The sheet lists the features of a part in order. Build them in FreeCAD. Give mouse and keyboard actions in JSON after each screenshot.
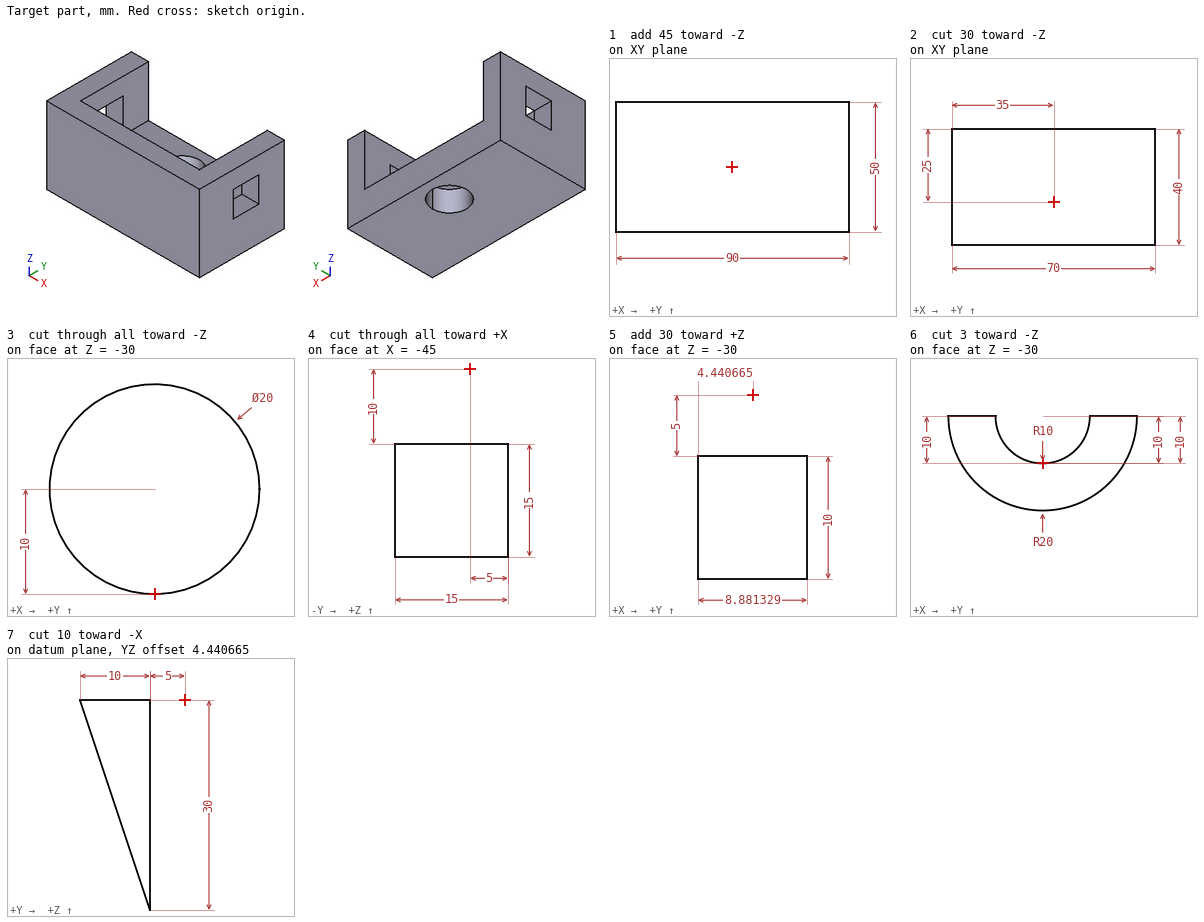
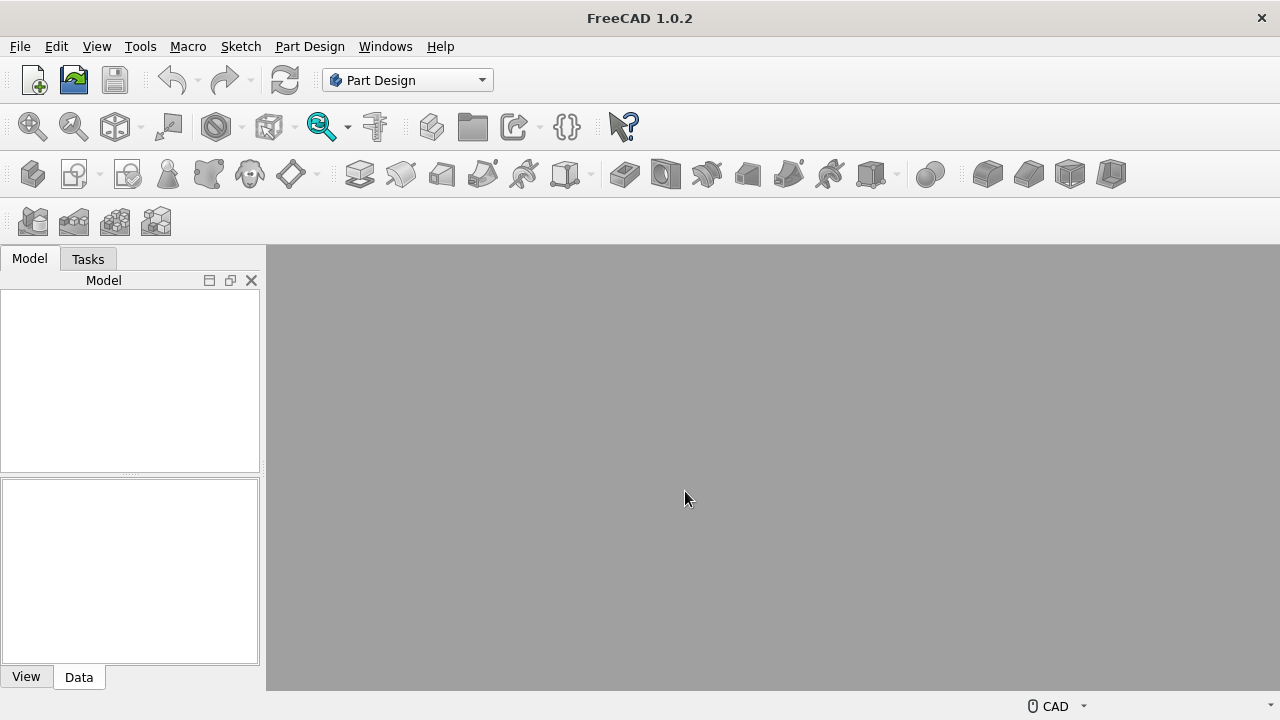
{"action": "key", "text": "ctrl+n"}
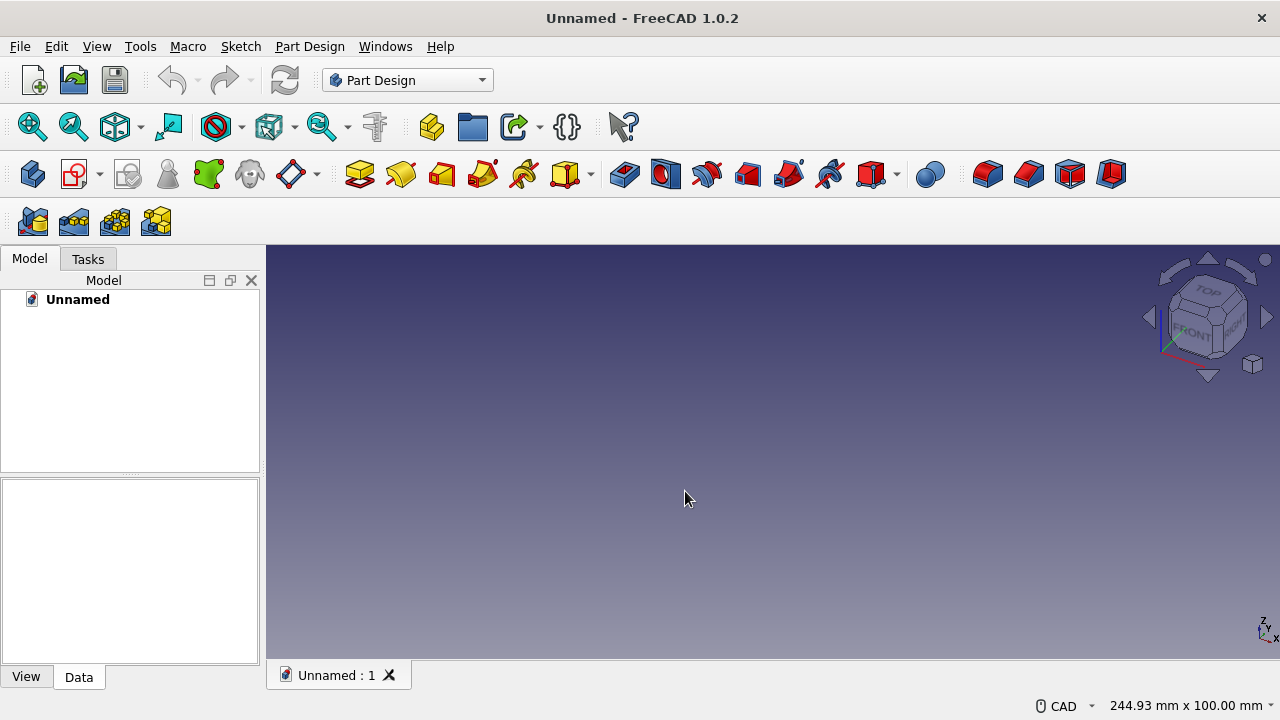
{"action": "left_click", "coordinate": [74, 174]}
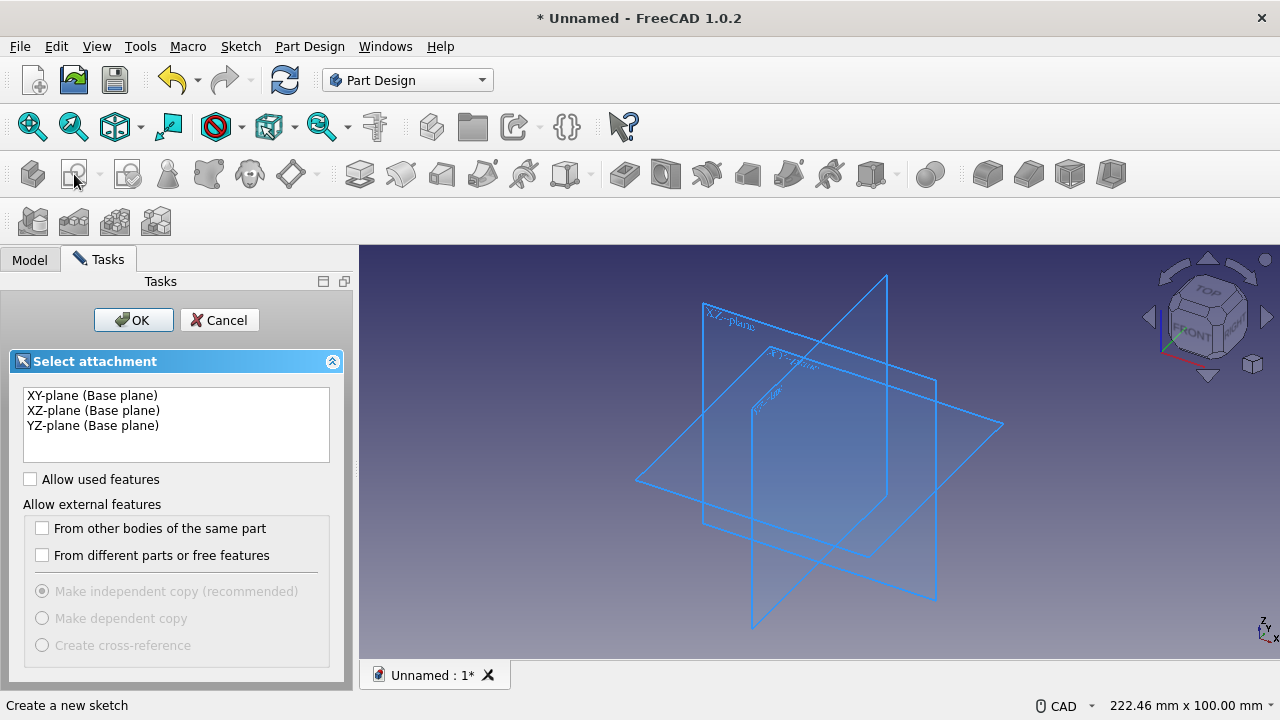
{"action": "left_click", "coordinate": [84, 396]}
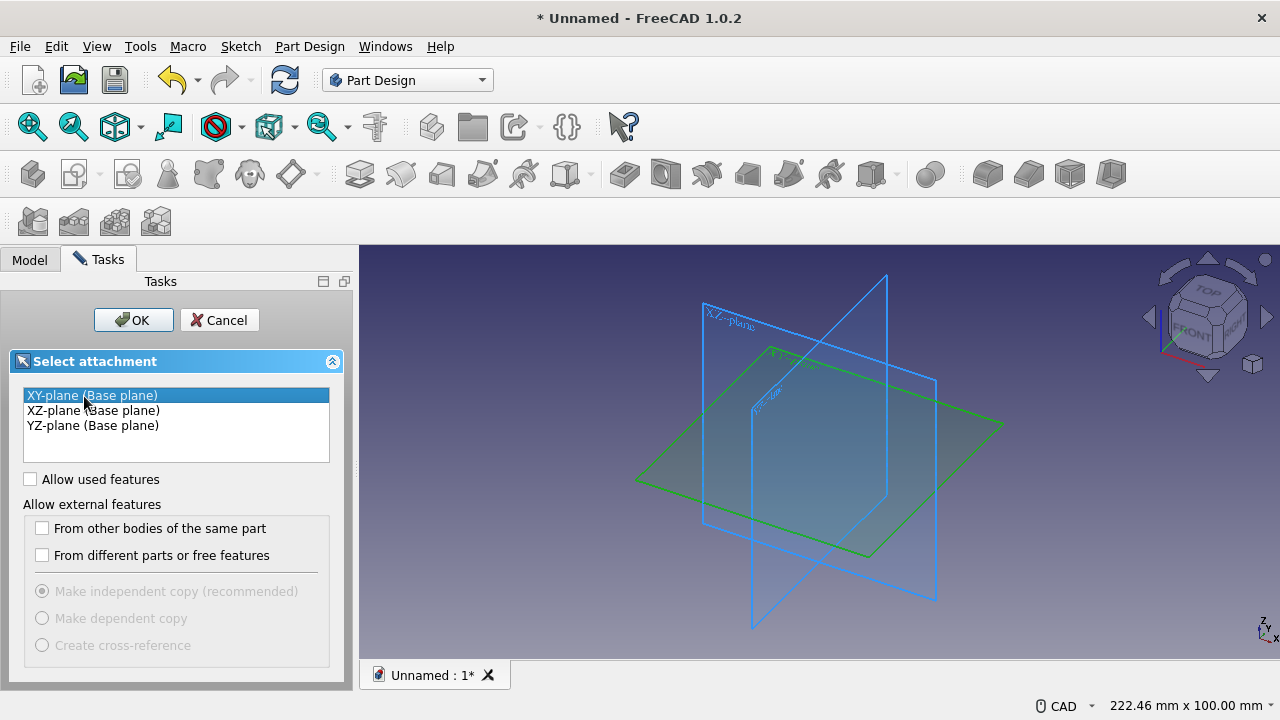
{"action": "left_click", "coordinate": [134, 320]}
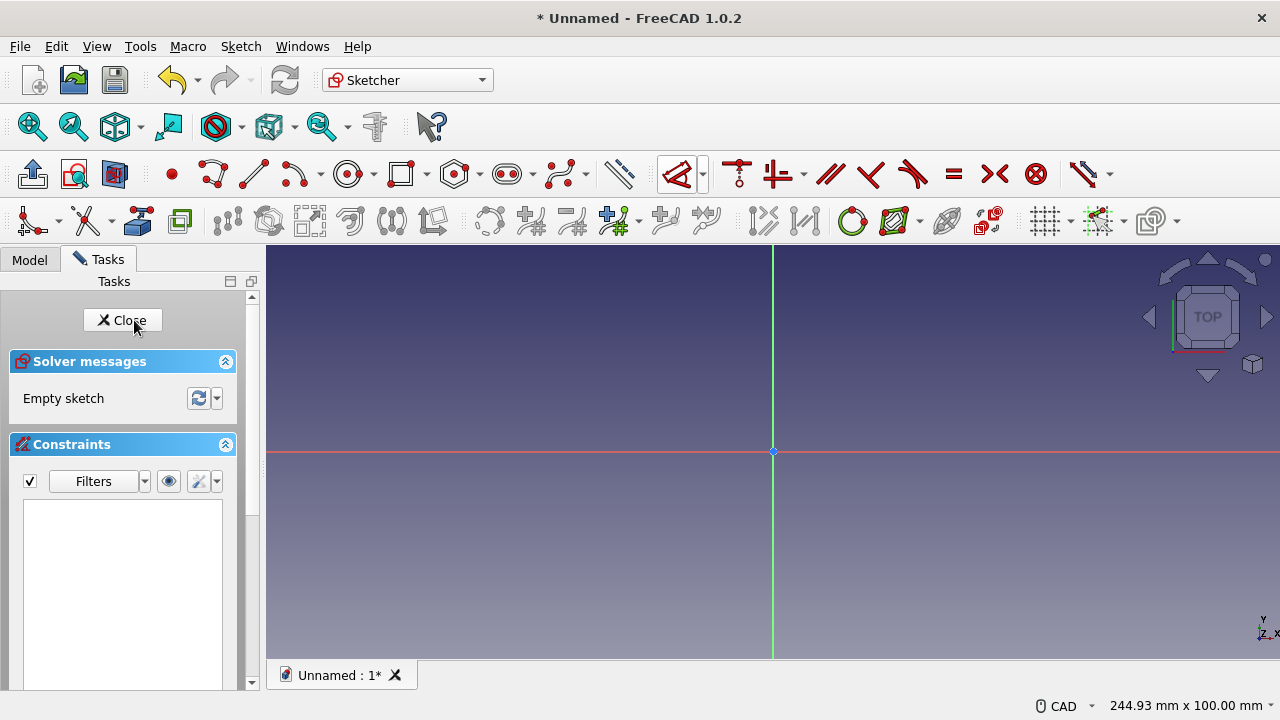
{"action": "key", "text": "g v"}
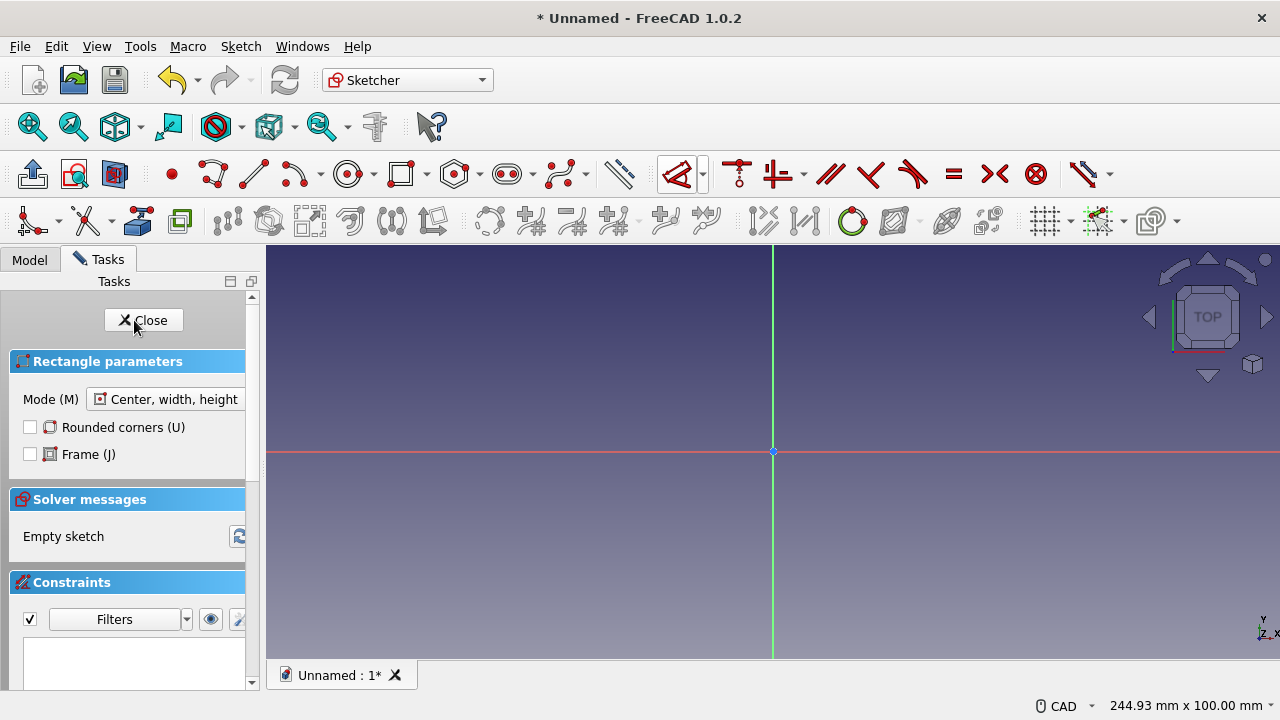
{"action": "left_click", "coordinate": [773, 452]}
{"action": "mouse_move", "coordinate": [959, 348]}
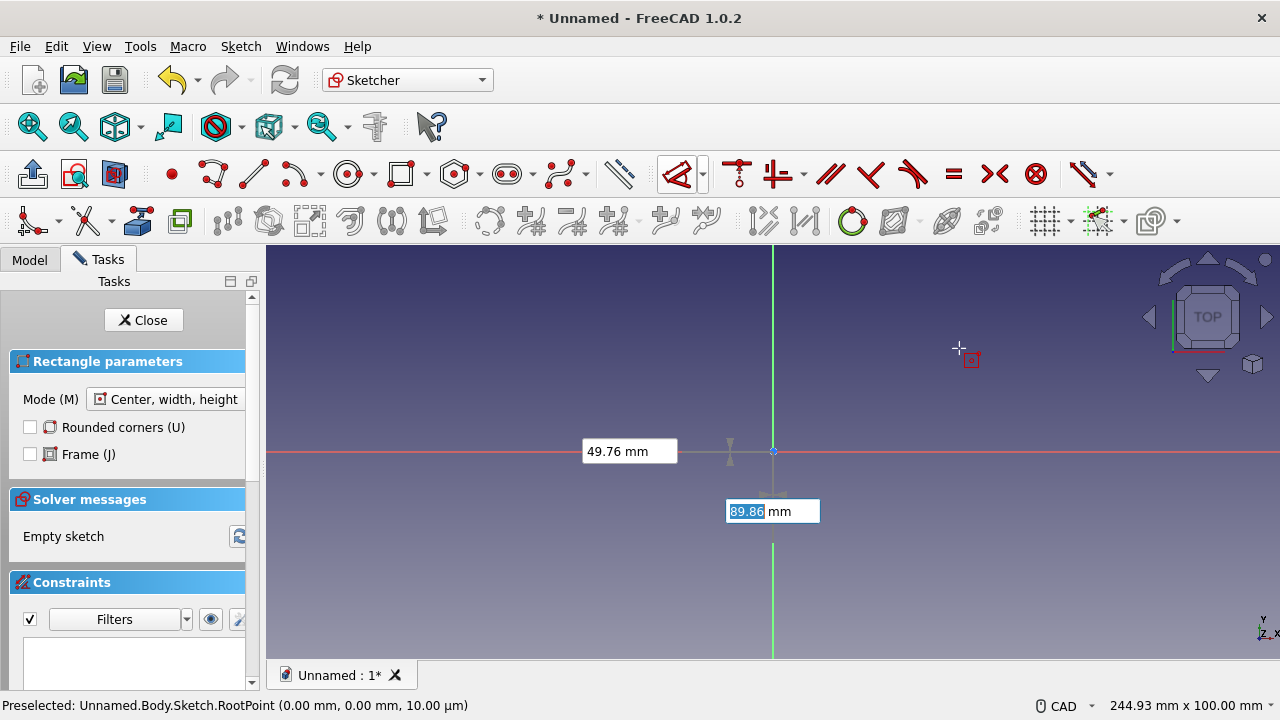
{"action": "type", "text": "90"}
{"action": "key", "text": "Tab"}
{"action": "type", "text": "50"}
{"action": "key", "text": "Return"}
{"action": "key", "text": "Escape"}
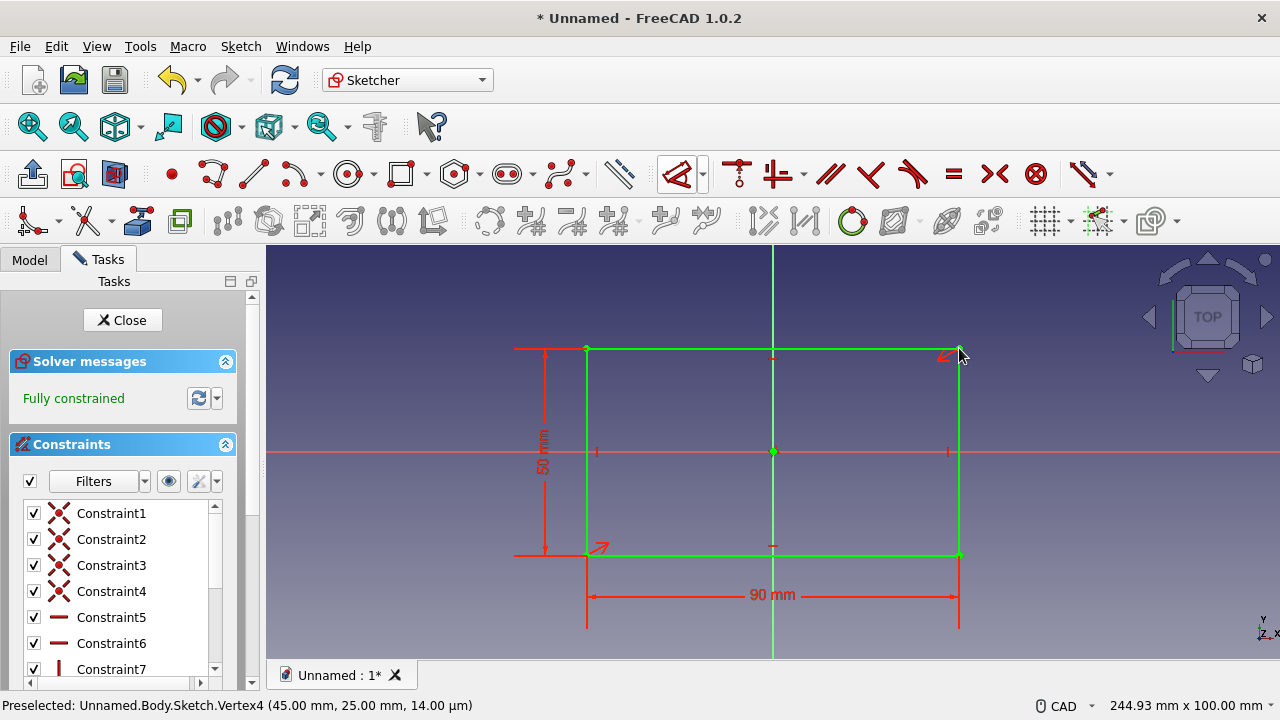
{"action": "left_click", "coordinate": [123, 320]}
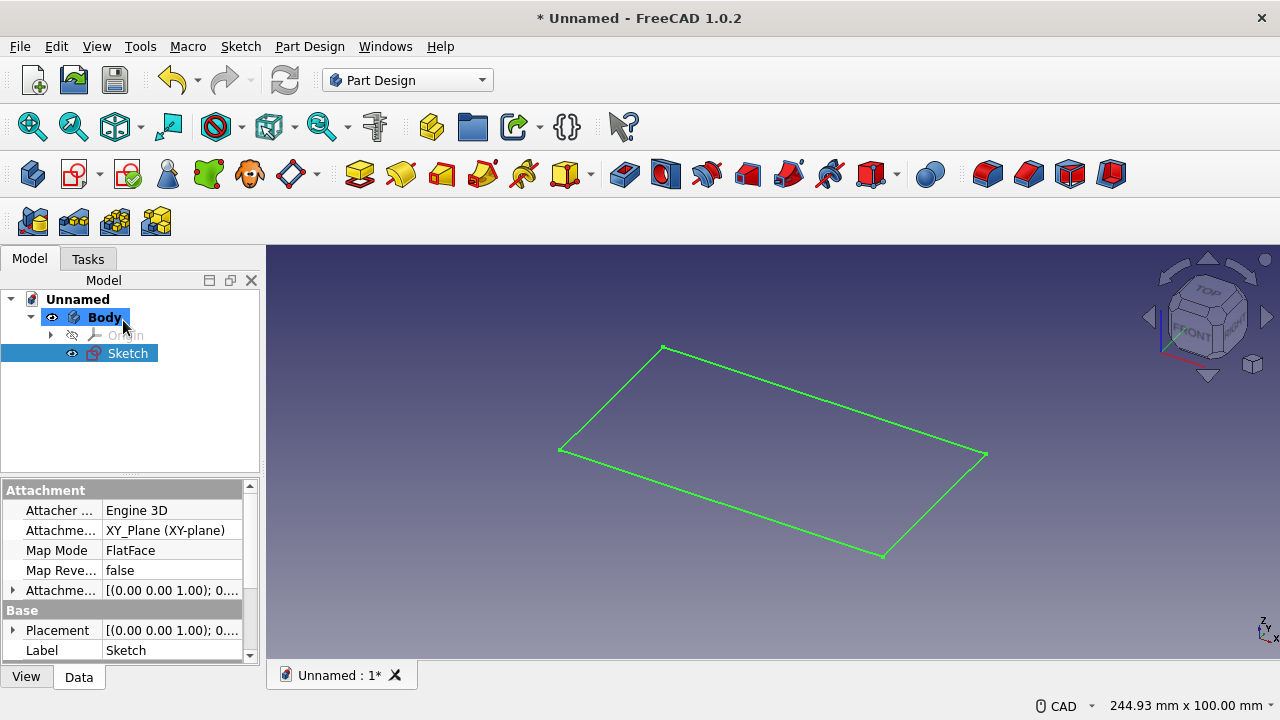
{"action": "left_click", "coordinate": [360, 174]}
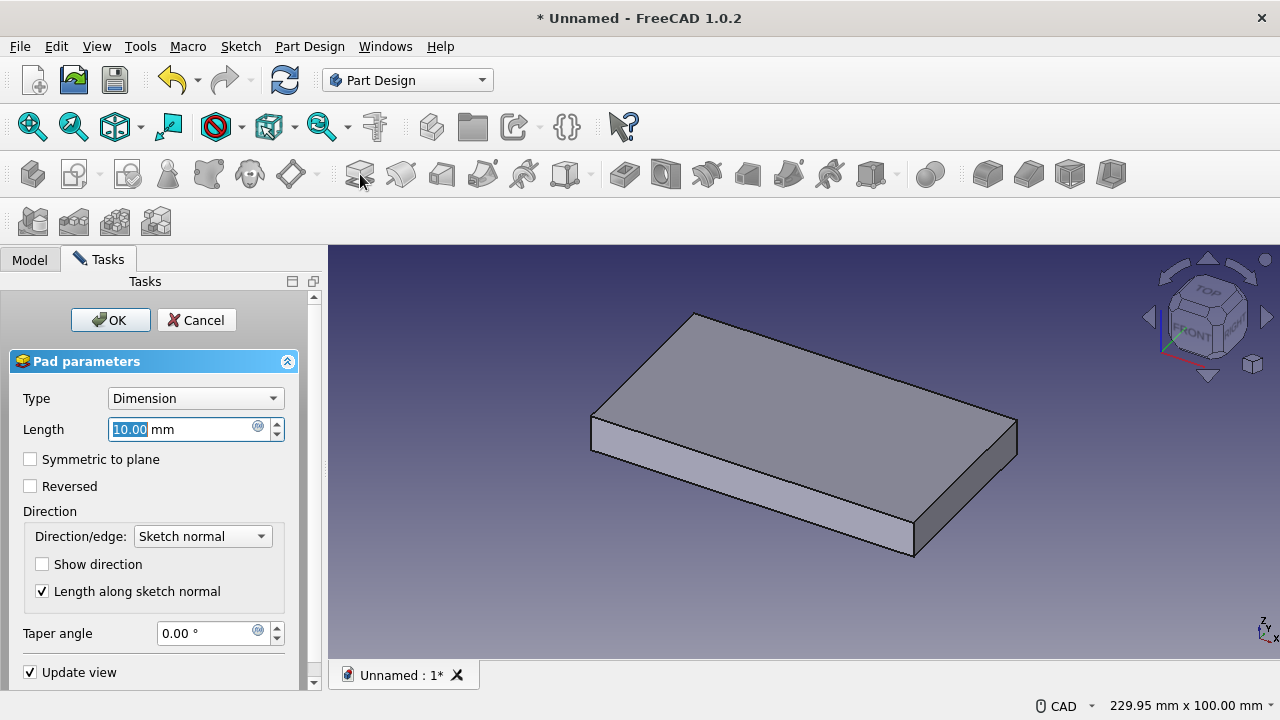
{"action": "type", "text": "45"}
{"action": "key", "text": "Tab"}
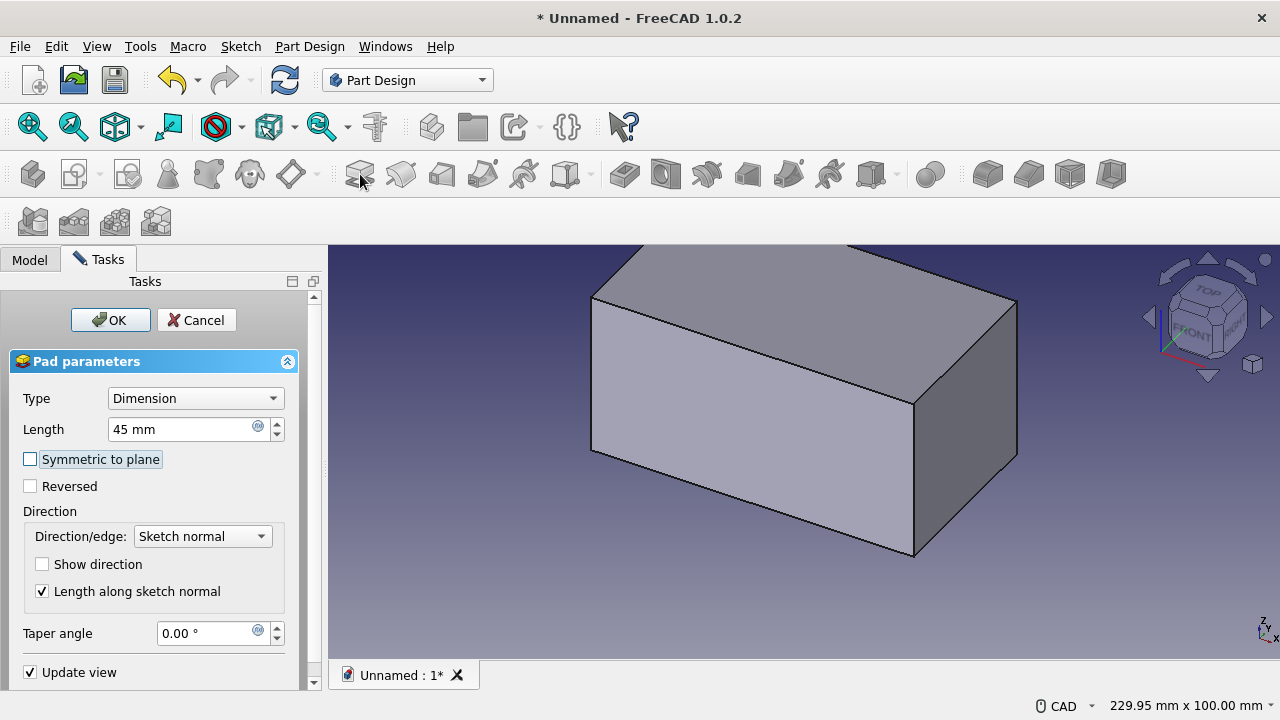
{"action": "left_click", "coordinate": [31, 486]}